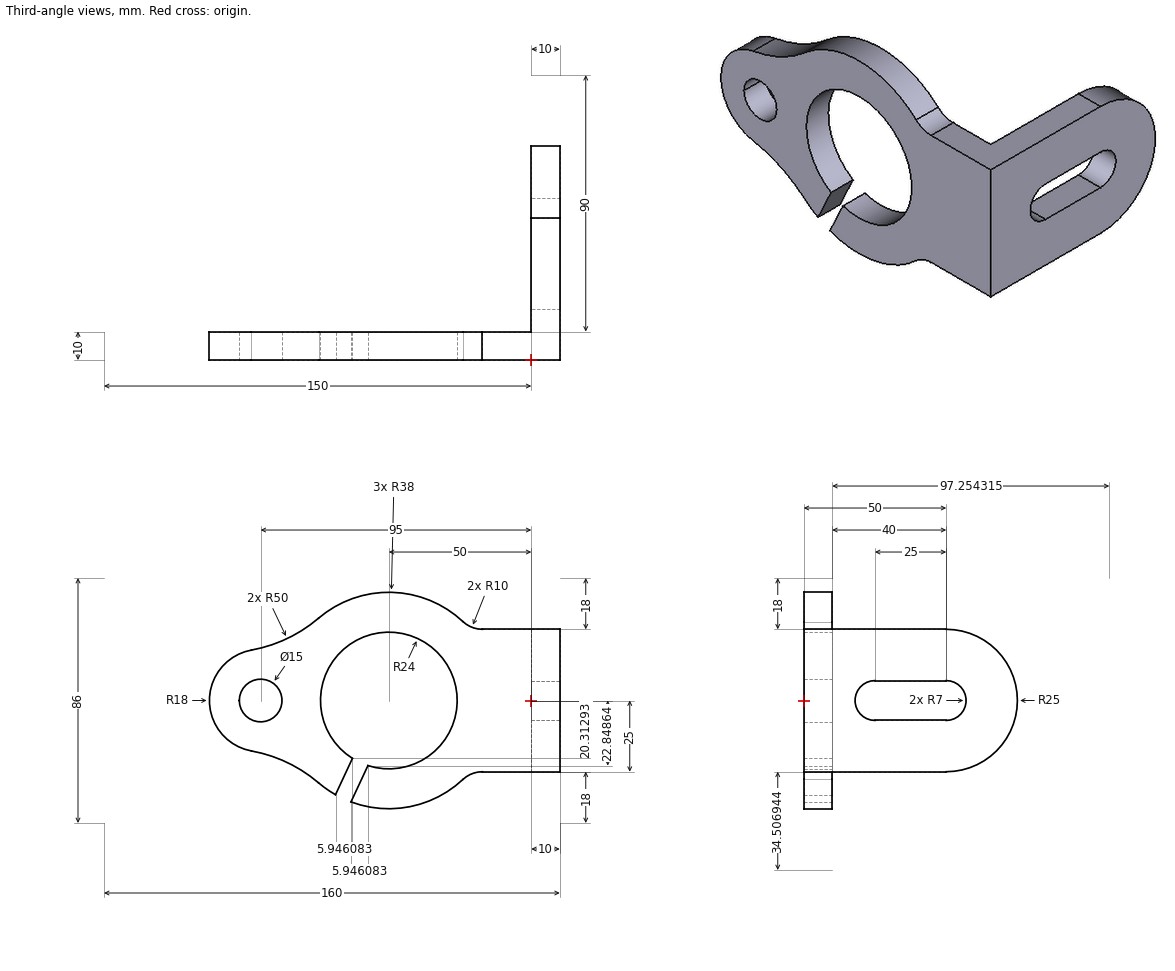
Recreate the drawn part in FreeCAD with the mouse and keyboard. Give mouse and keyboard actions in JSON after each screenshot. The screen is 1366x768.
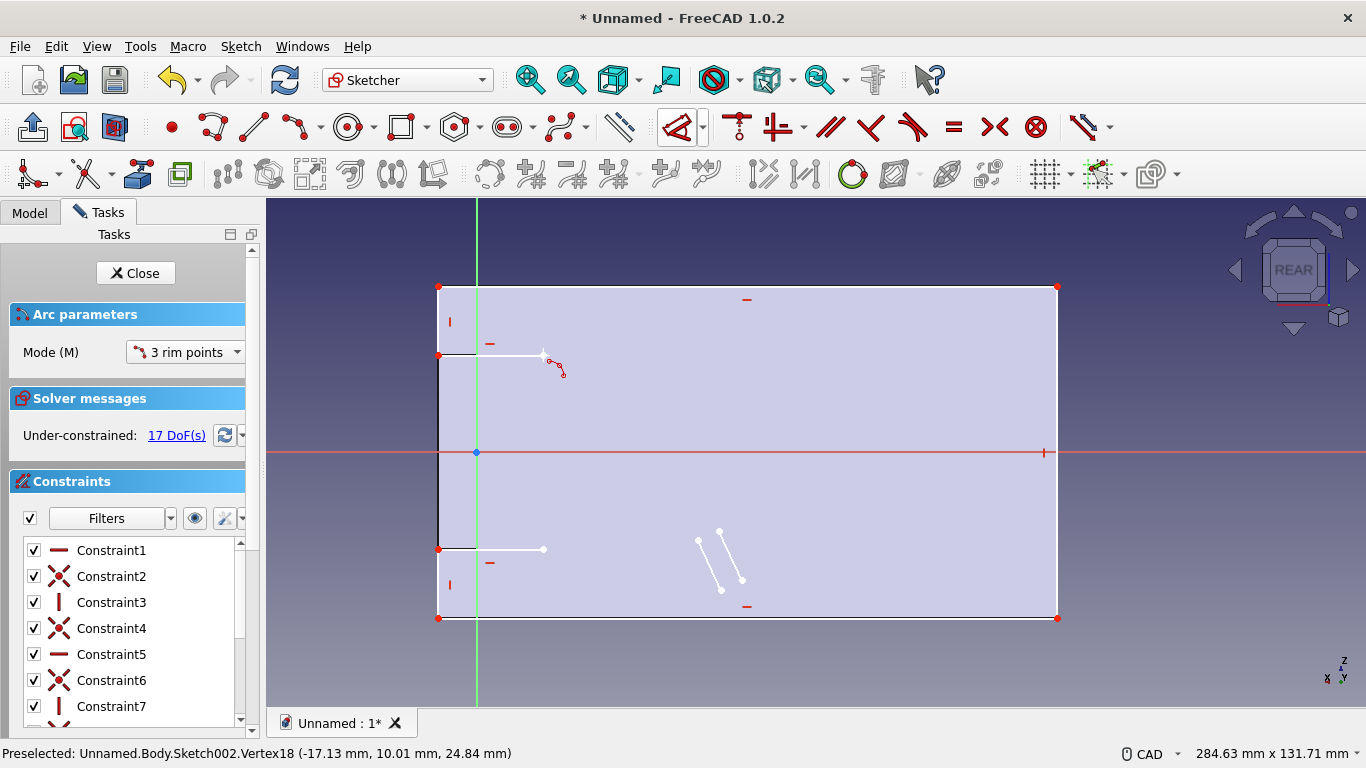
{"action": "left_click", "coordinate": [719, 532]}
{"action": "left_click", "coordinate": [698, 541]}
{"action": "left_click", "coordinate": [631, 368]}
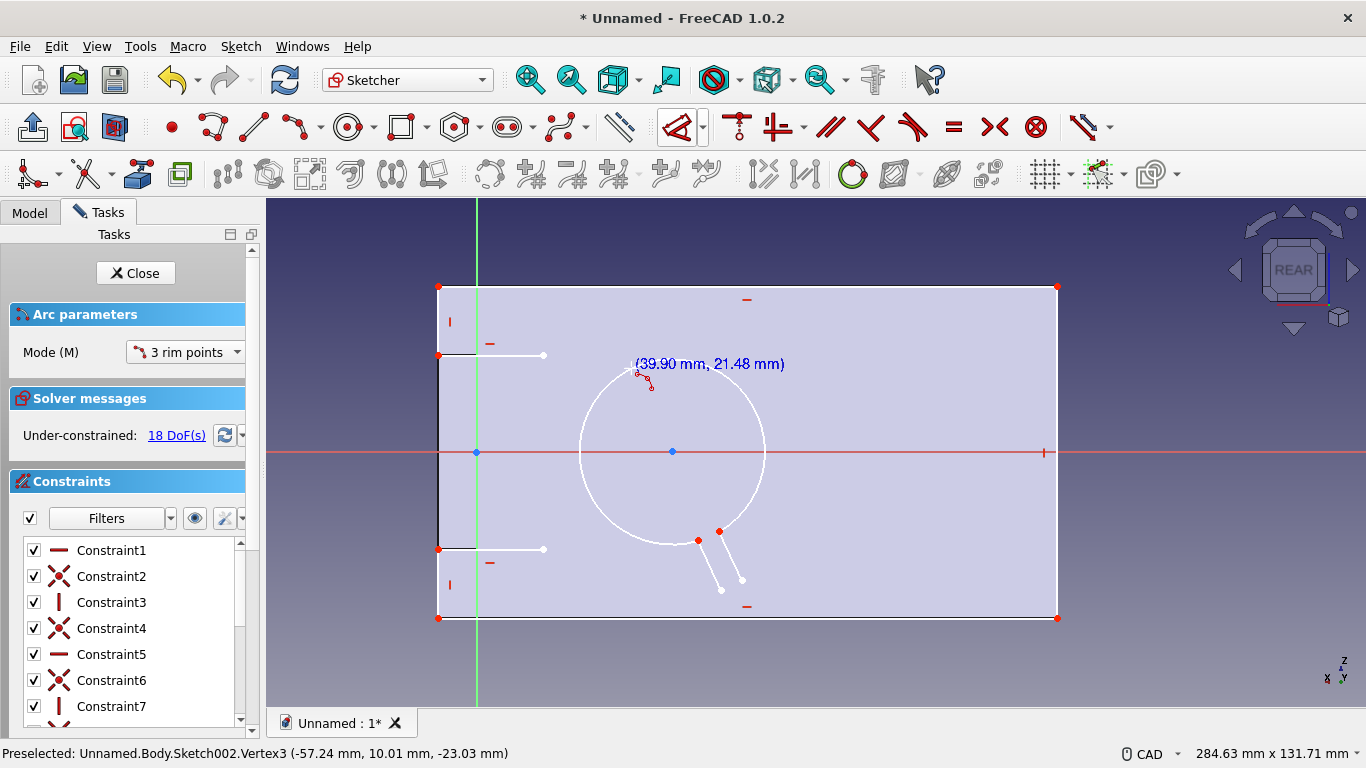
{"action": "left_click", "coordinate": [721, 591]}
{"action": "left_click", "coordinate": [570, 559]}
{"action": "left_click", "coordinate": [641, 596]}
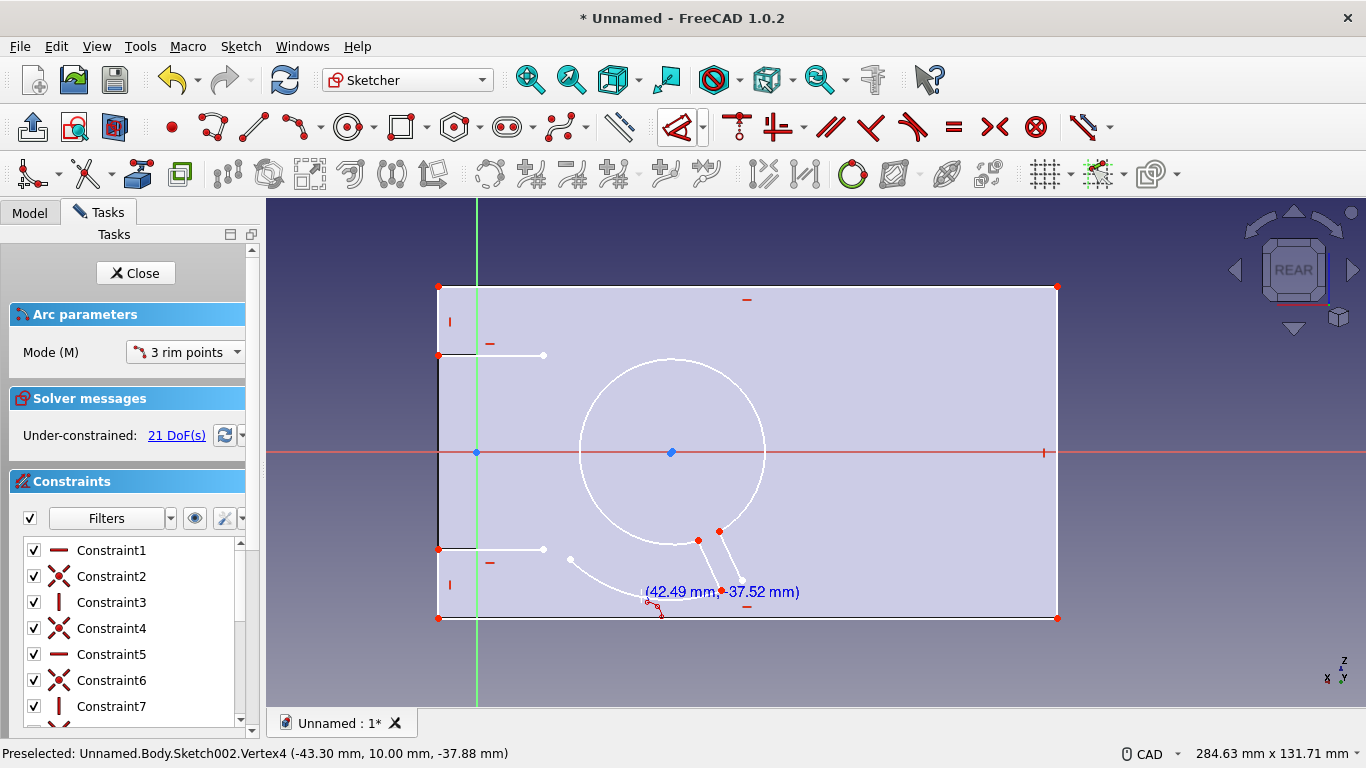
{"action": "left_click", "coordinate": [570, 560]}
{"action": "left_click", "coordinate": [543, 550]}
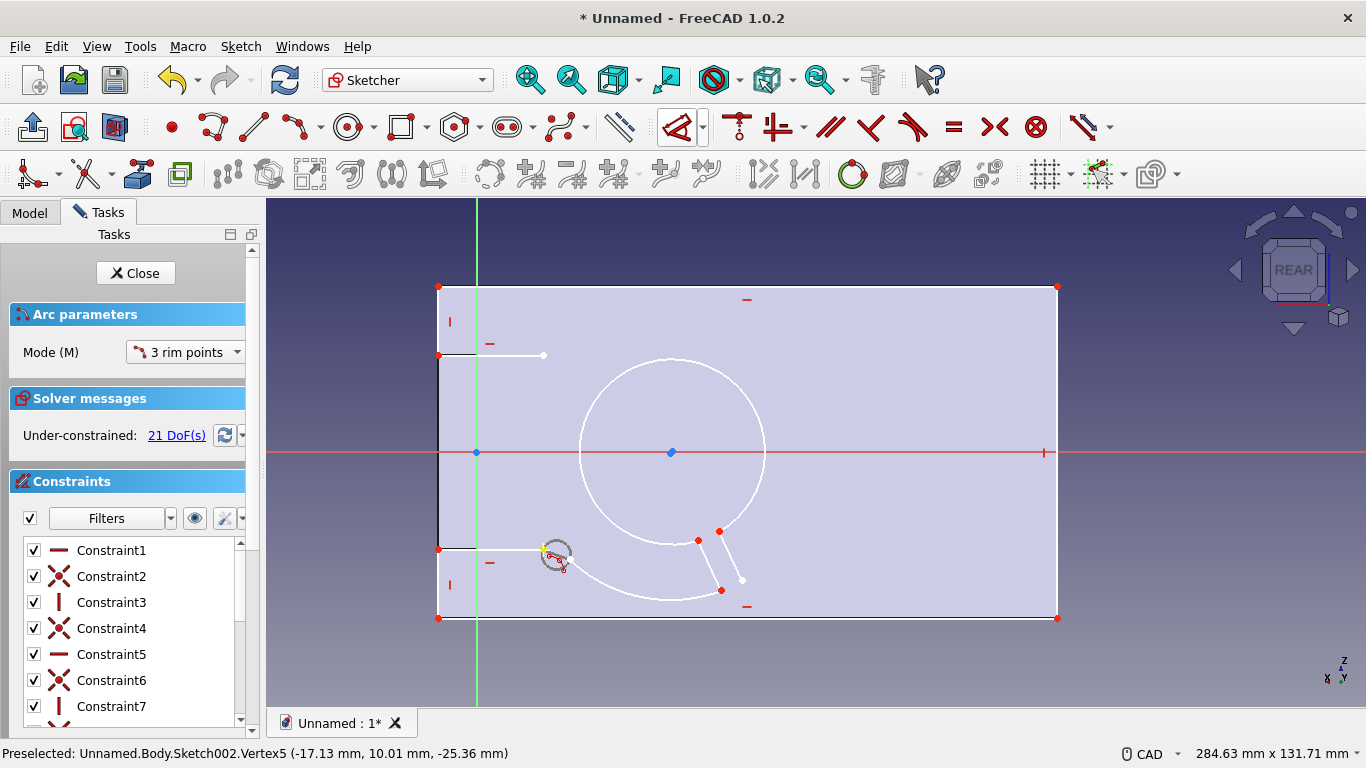
{"action": "scroll", "coordinate": [557, 551], "scroll_direction": "up", "scroll_amount": 9}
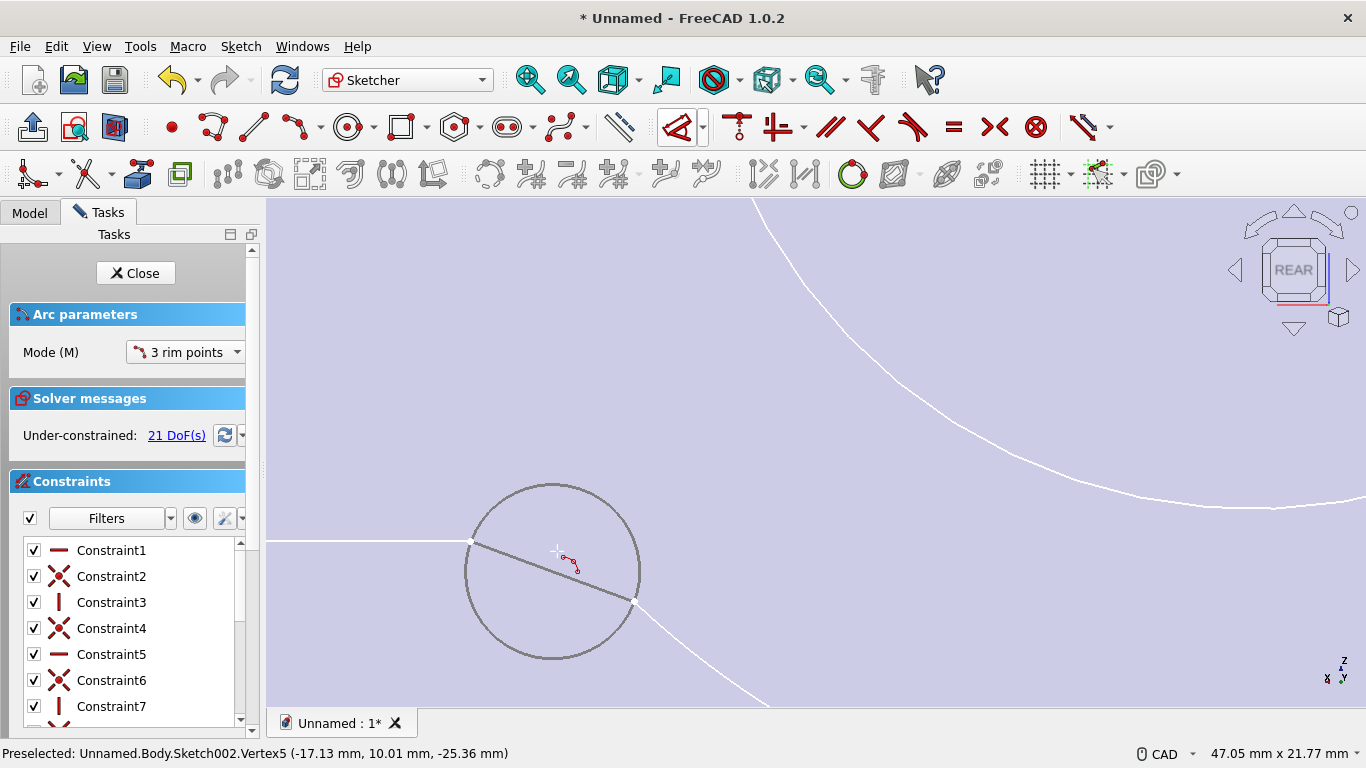
{"action": "left_click", "coordinate": [558, 550]}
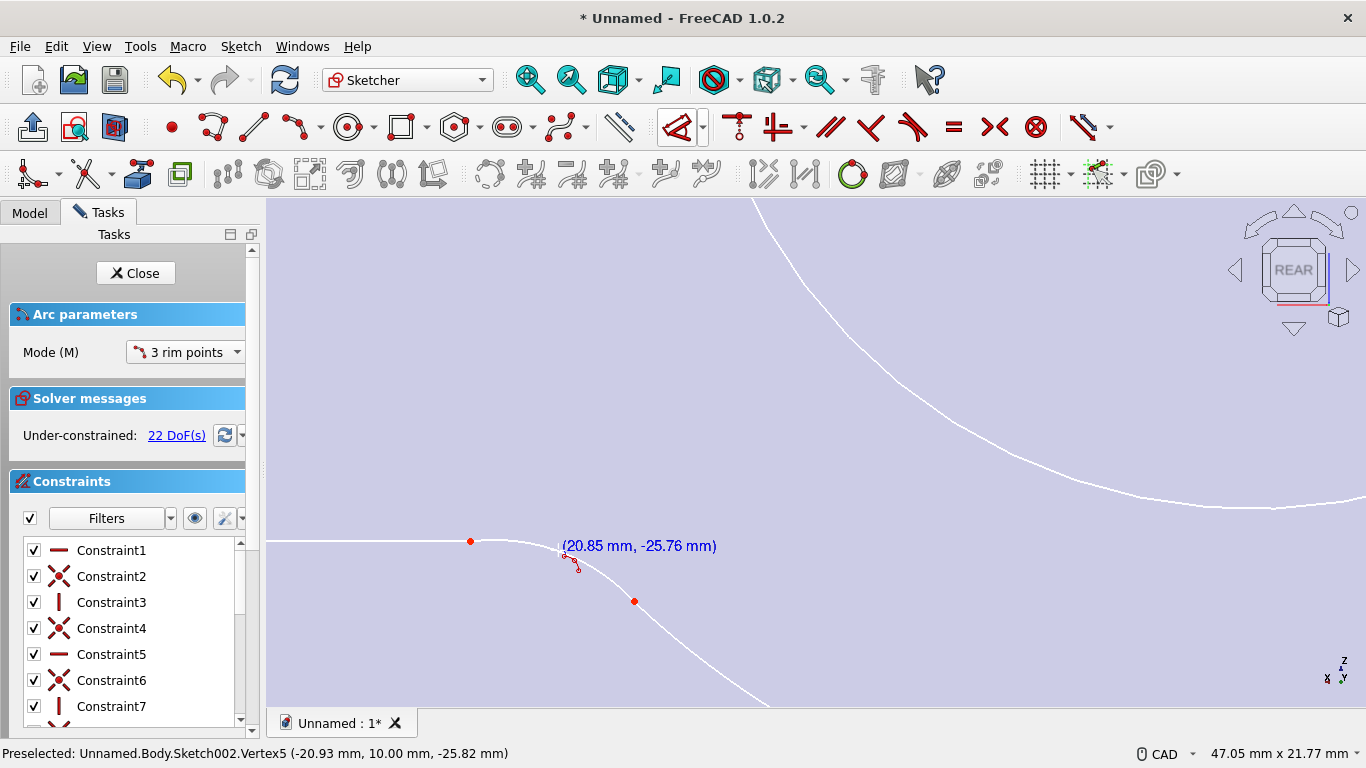
{"action": "scroll", "coordinate": [557, 552], "scroll_direction": "down", "scroll_amount": 9}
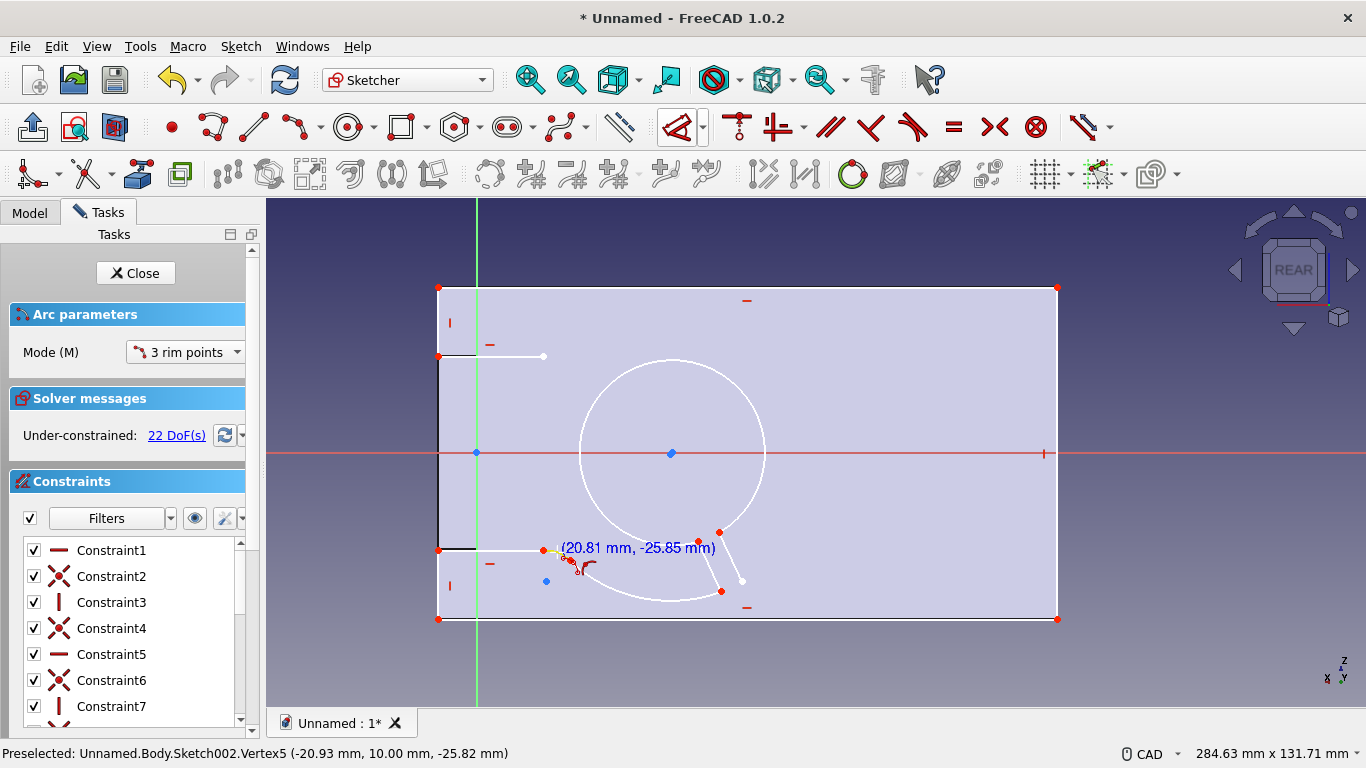
{"action": "left_click", "coordinate": [543, 357]}
{"action": "left_click", "coordinate": [570, 346]}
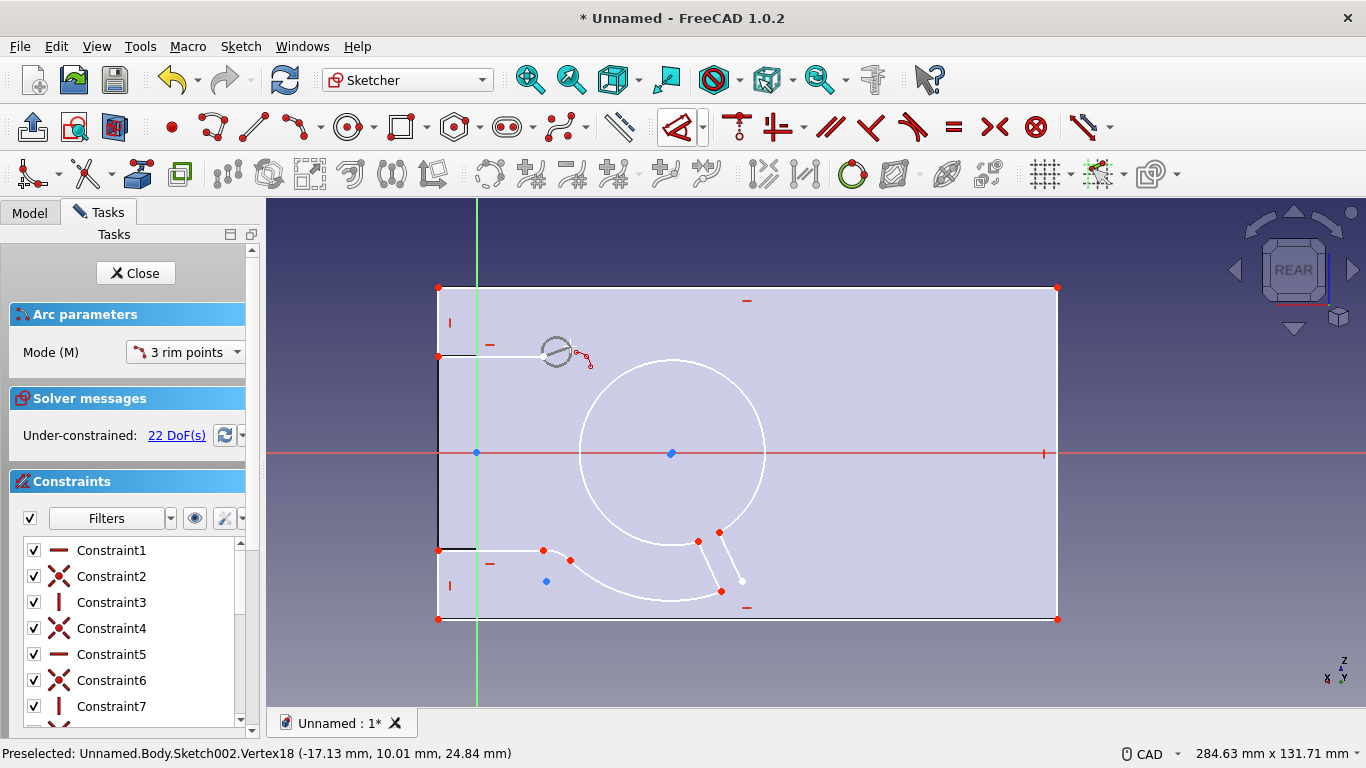
{"action": "scroll", "coordinate": [557, 354], "scroll_direction": "up", "scroll_amount": 9}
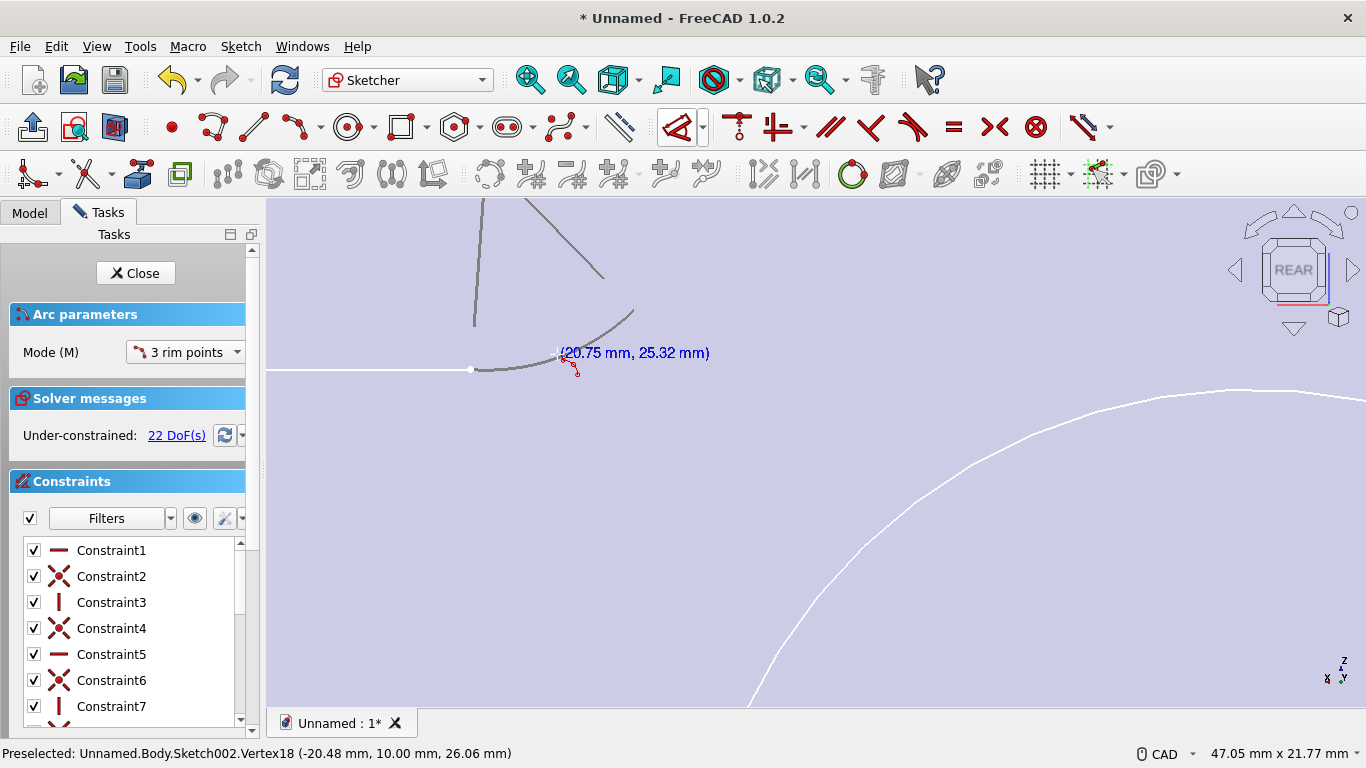
{"action": "left_click", "coordinate": [558, 350]}